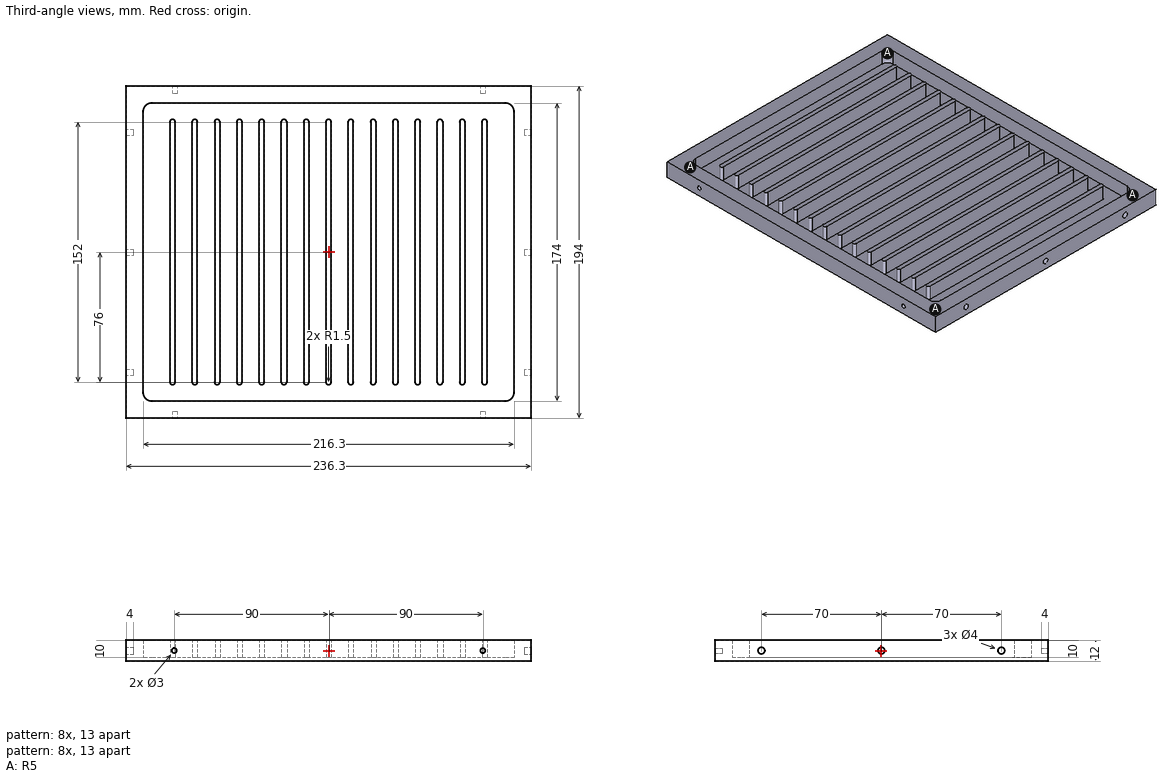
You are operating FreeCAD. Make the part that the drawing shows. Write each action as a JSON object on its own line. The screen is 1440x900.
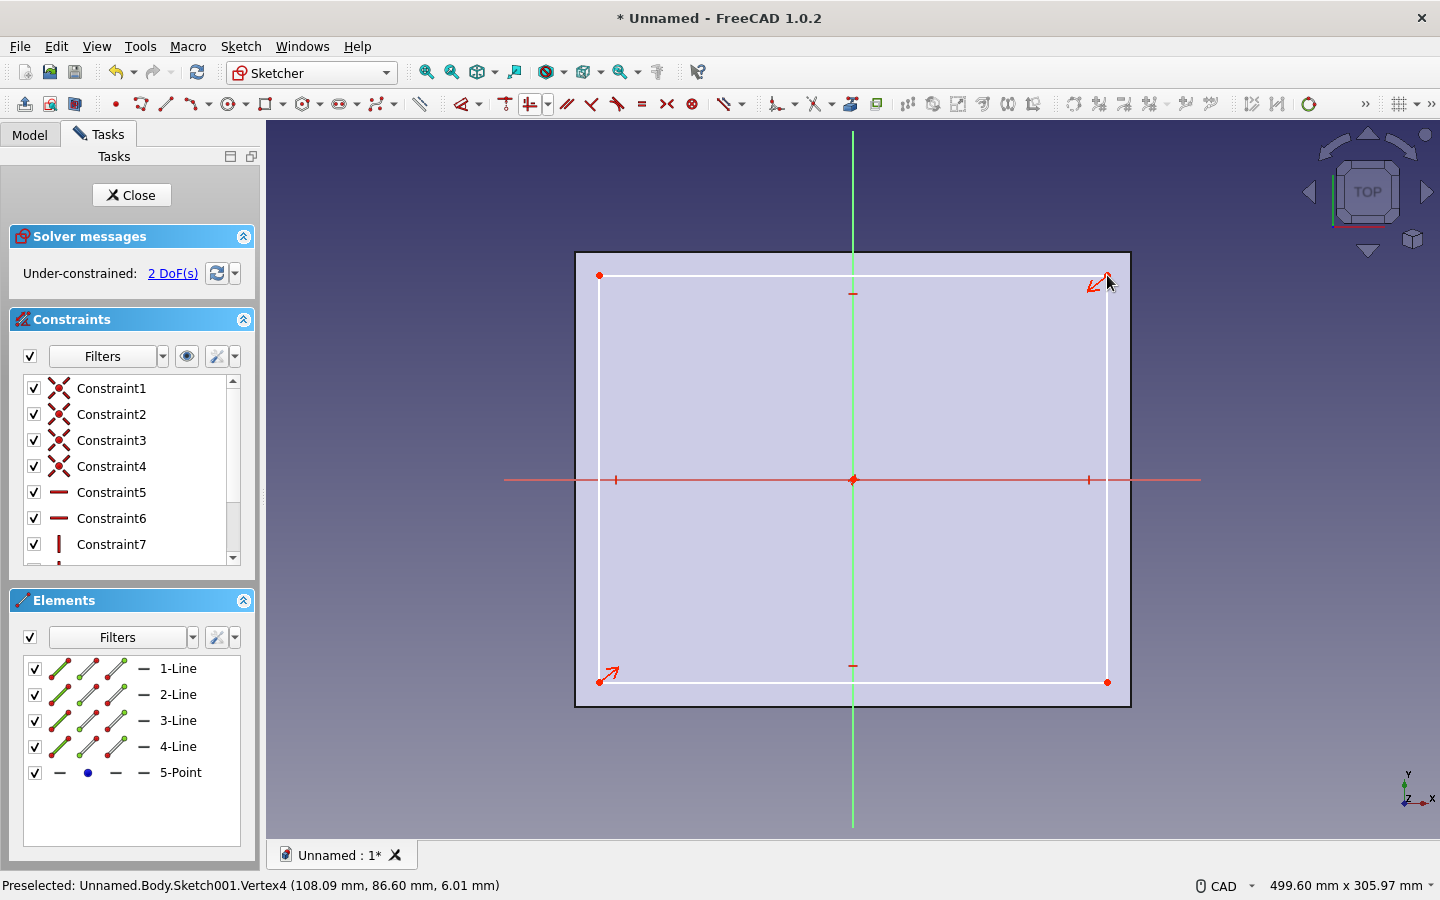
{"action": "left_click", "coordinate": [460, 104]}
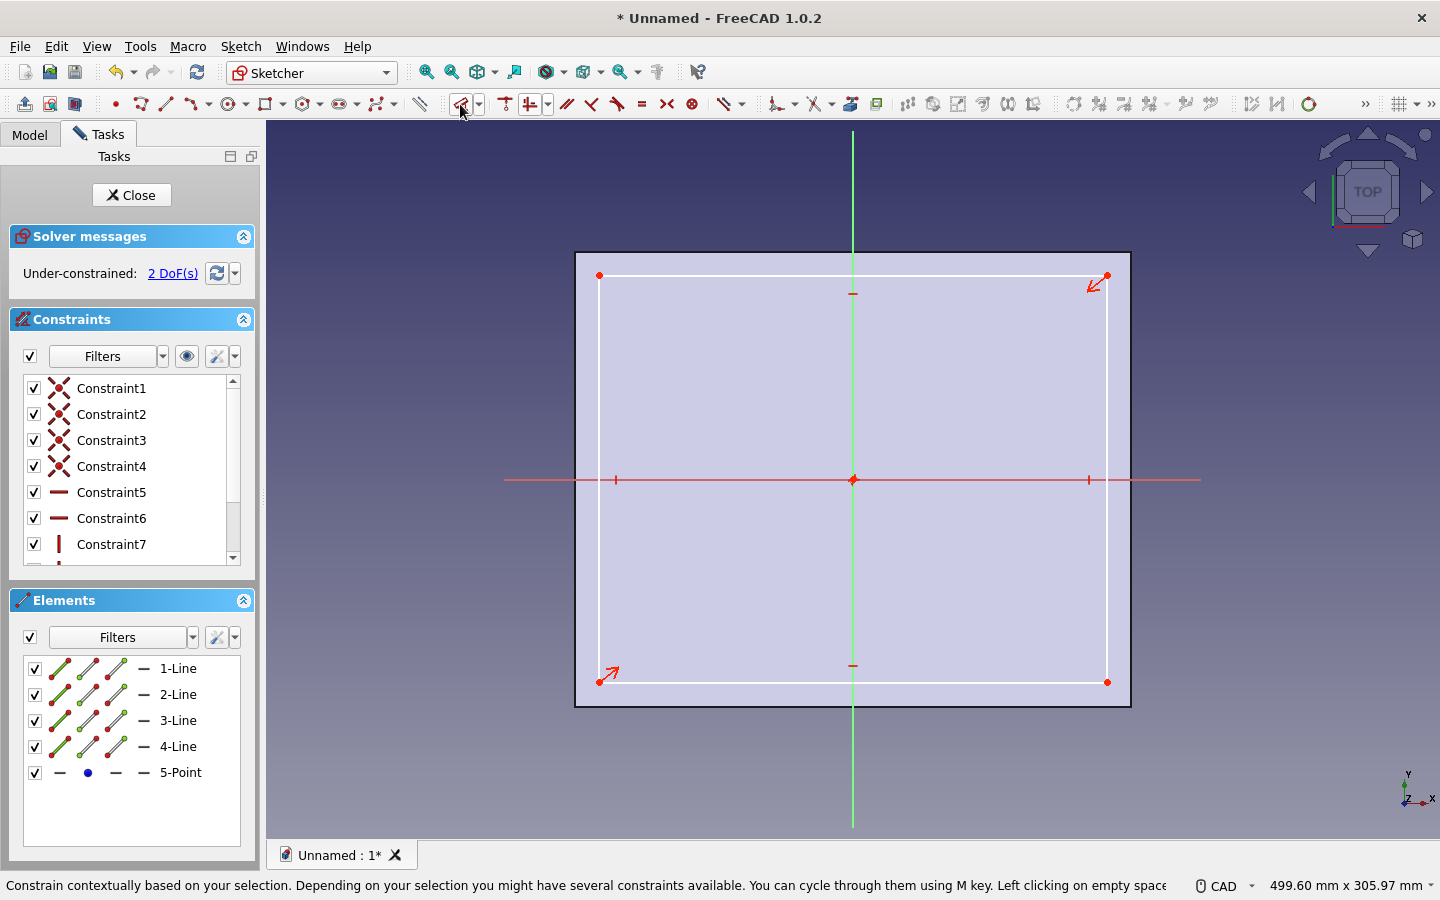
{"action": "left_click", "coordinate": [1107, 561]}
{"action": "left_click", "coordinate": [1141, 386]}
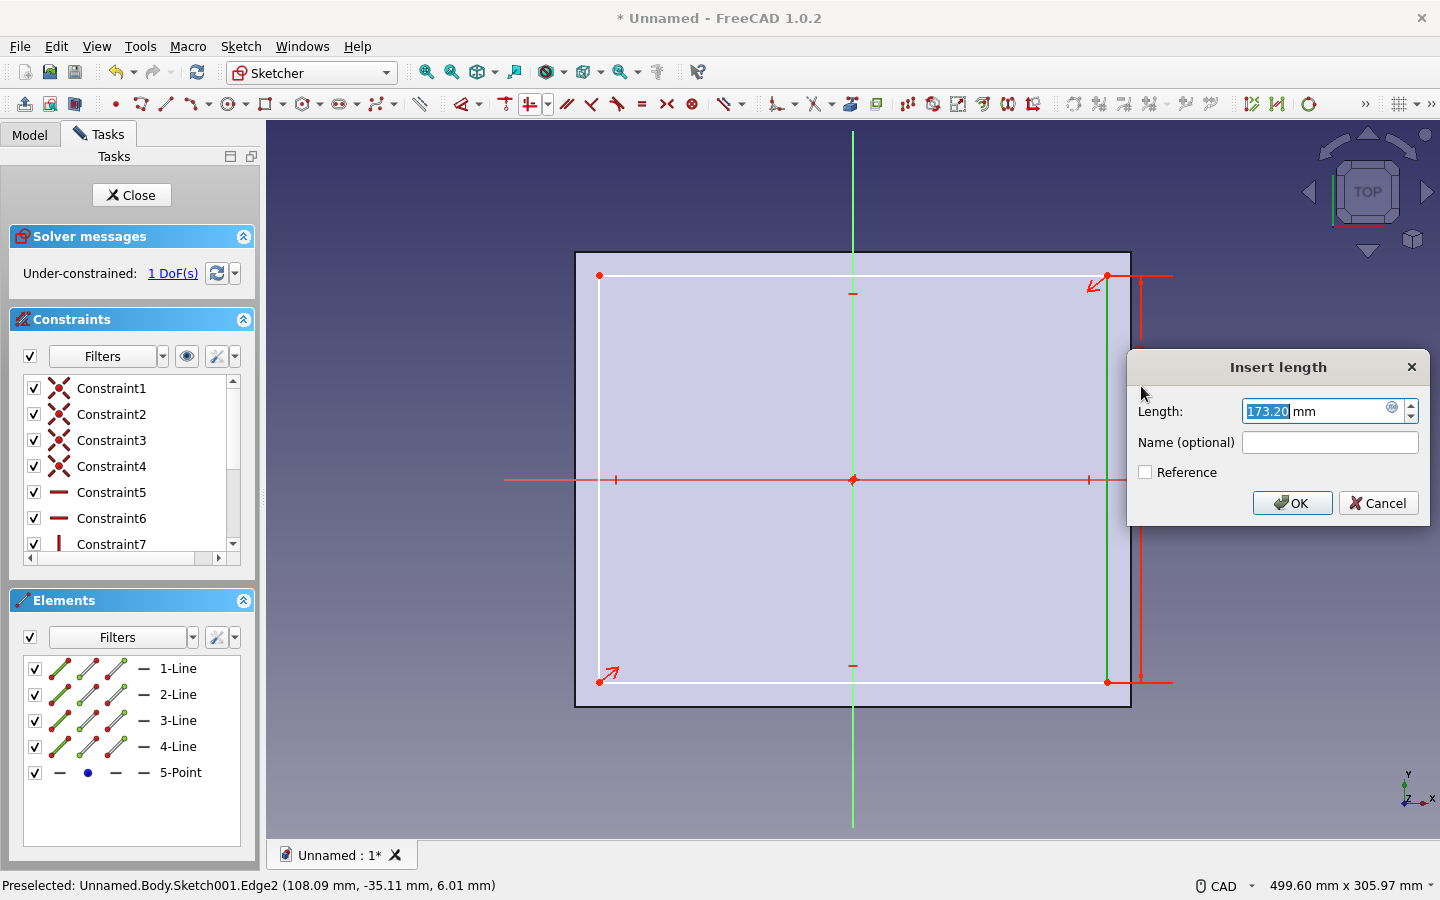
{"action": "type", "text": "174"}
{"action": "key", "text": "Return"}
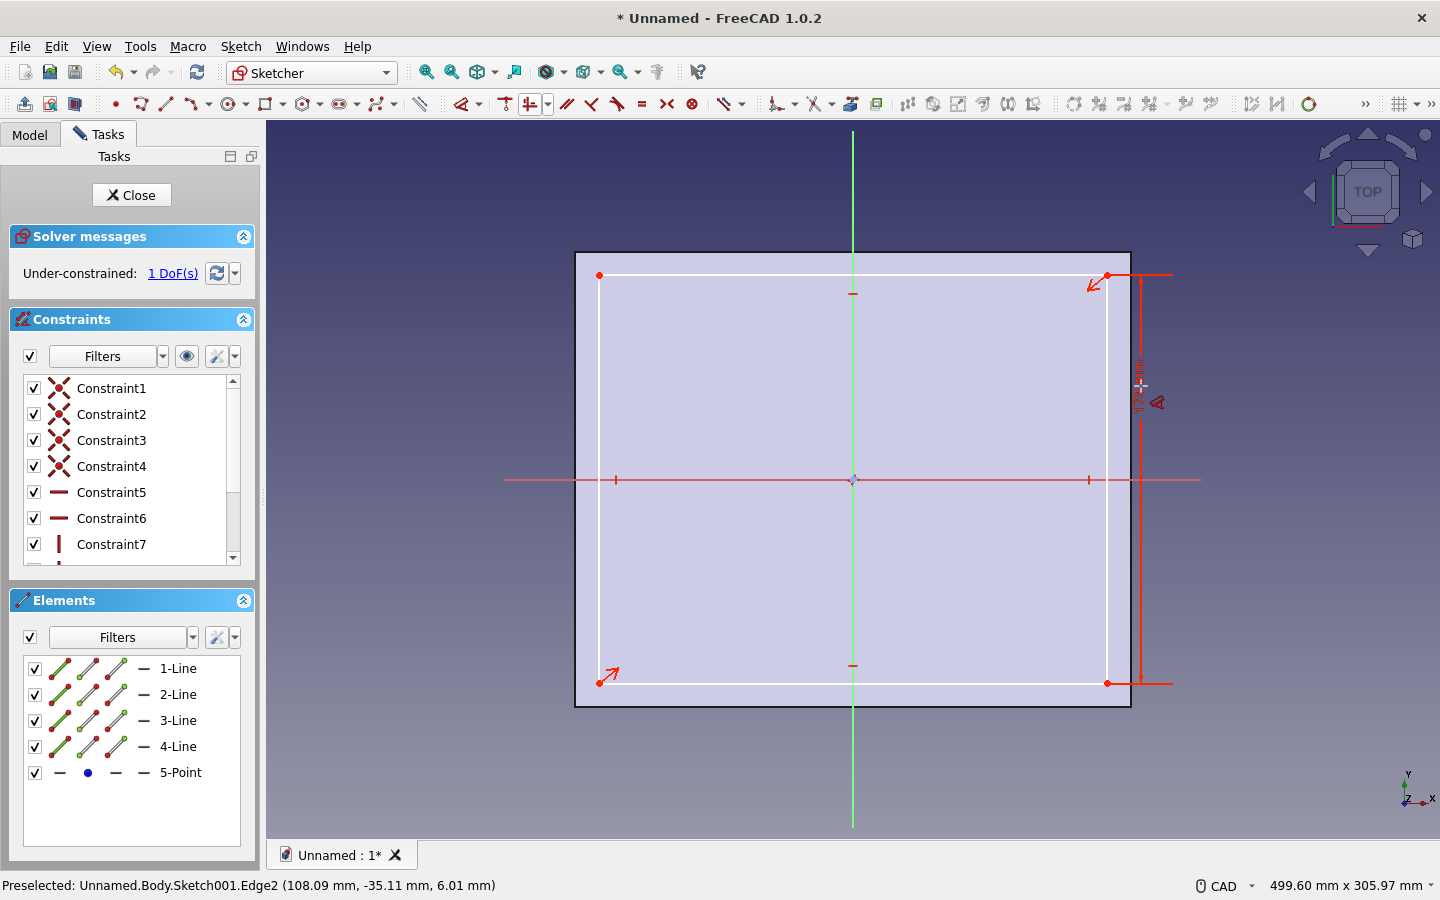
{"action": "left_click", "coordinate": [751, 684]}
{"action": "left_click", "coordinate": [736, 718]}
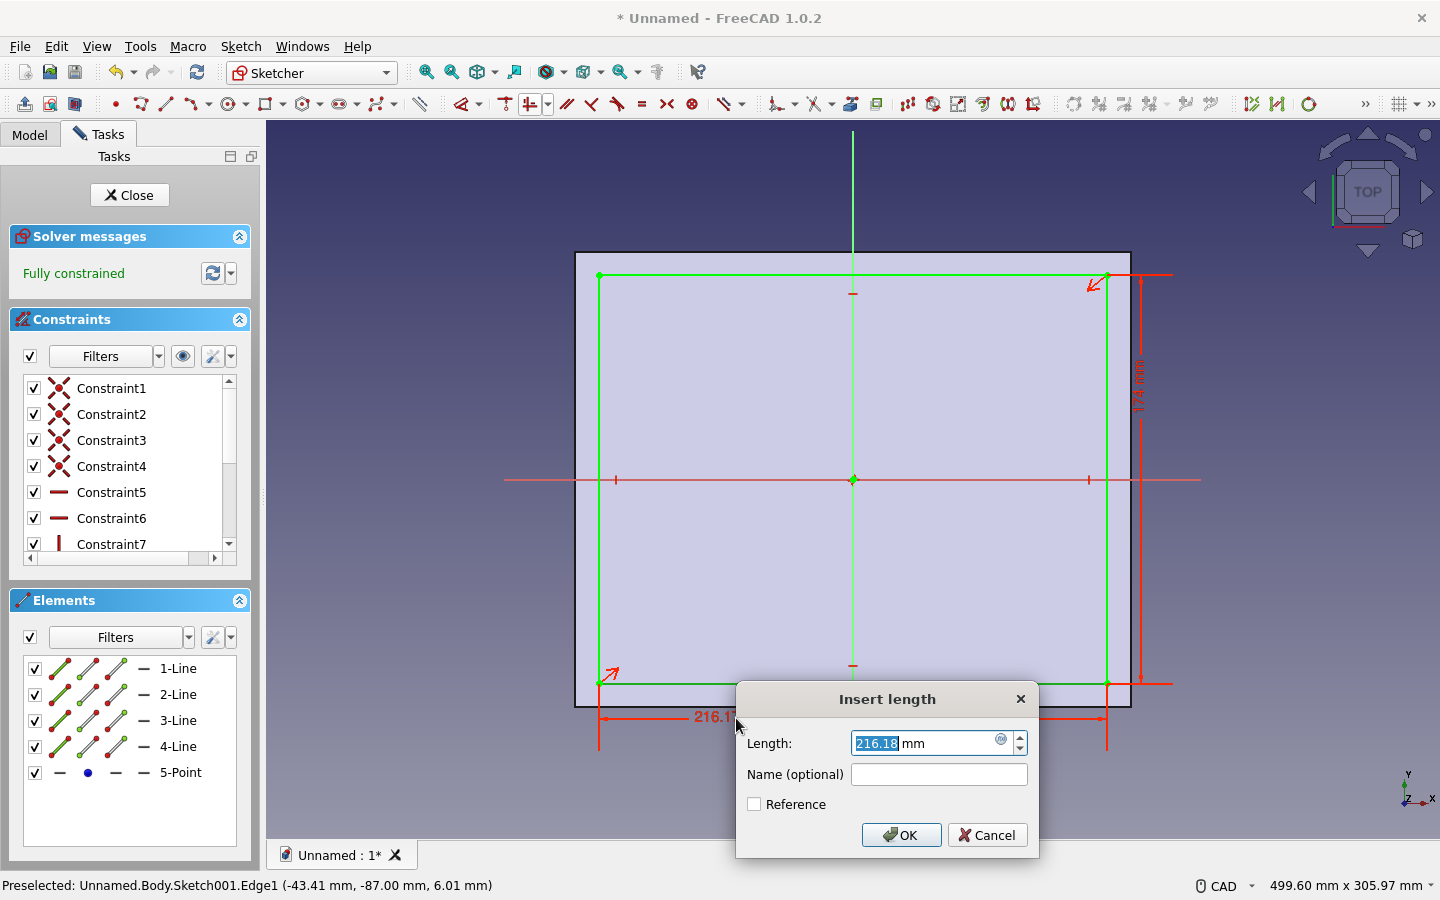
{"action": "type", "text": "216.3"}
{"action": "key", "text": "Return"}
{"action": "key", "text": "Escape"}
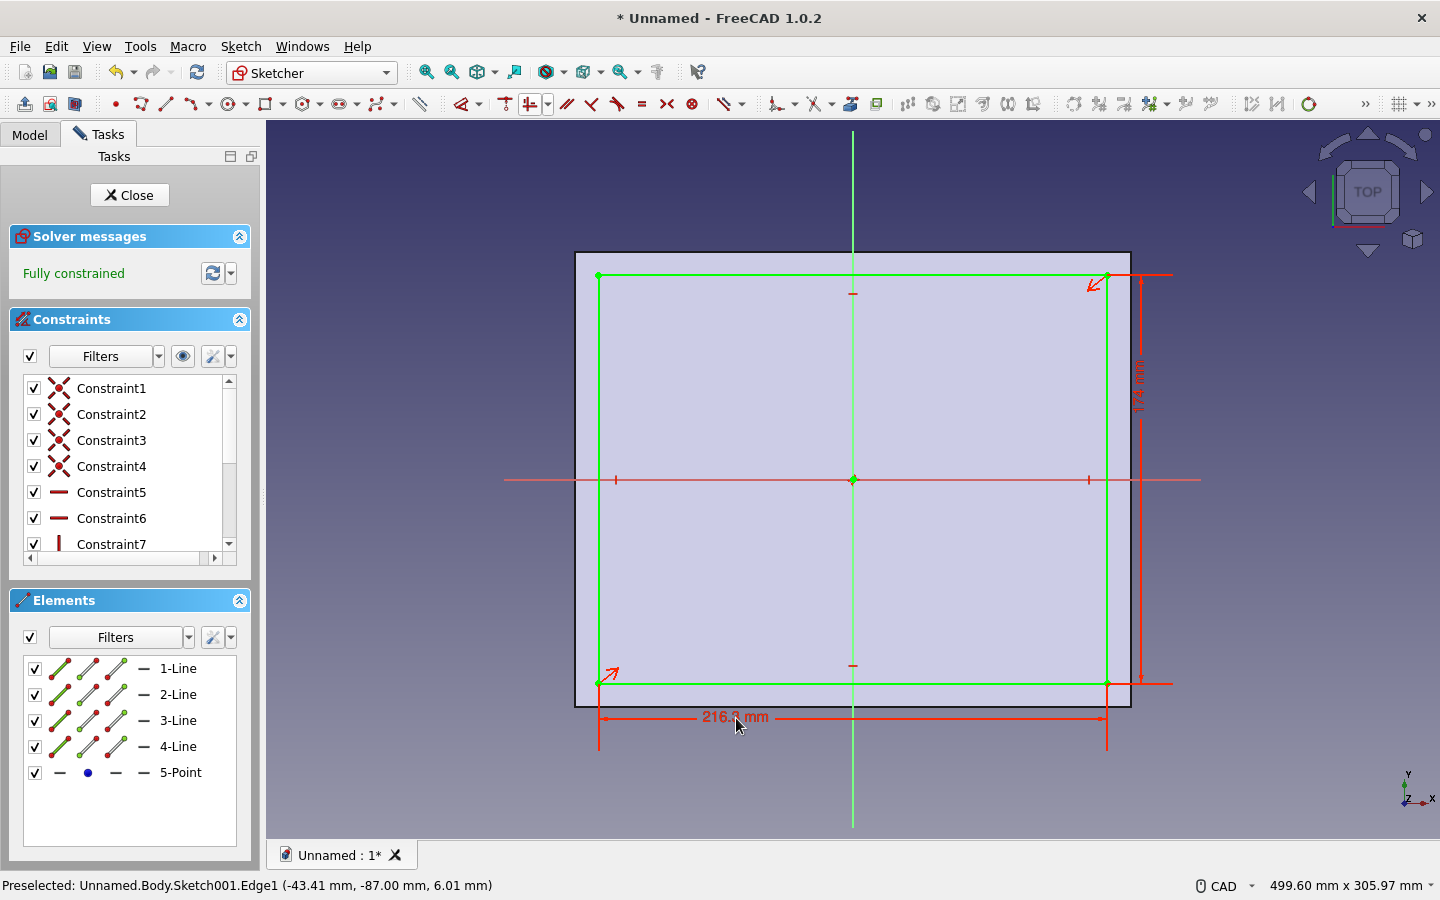
{"action": "left_click", "coordinate": [130, 195]}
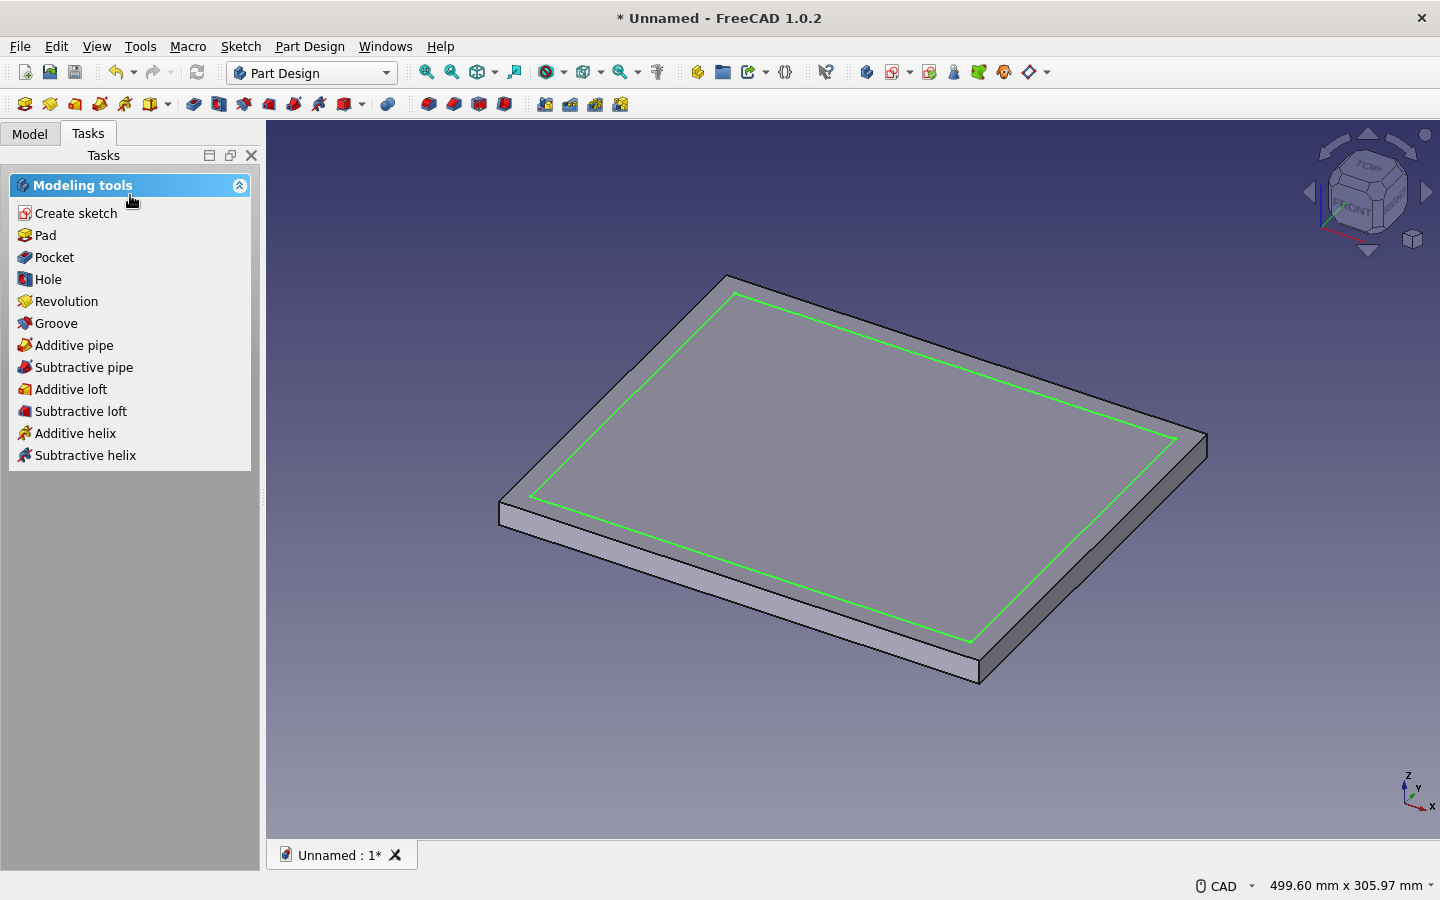
{"action": "left_click", "coordinate": [194, 104]}